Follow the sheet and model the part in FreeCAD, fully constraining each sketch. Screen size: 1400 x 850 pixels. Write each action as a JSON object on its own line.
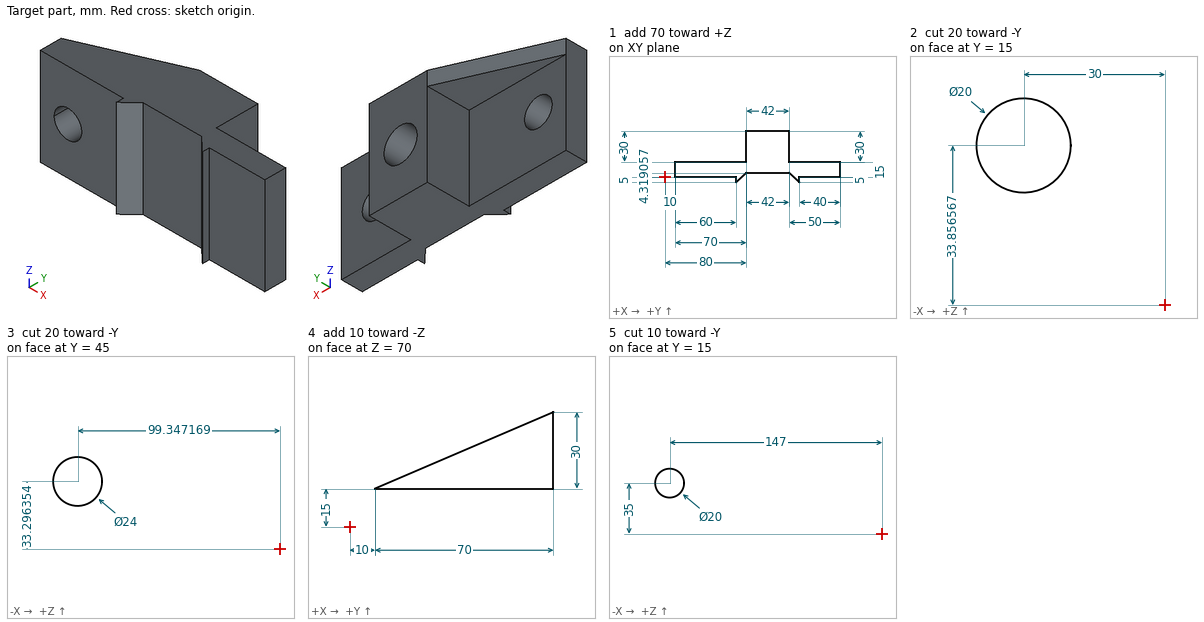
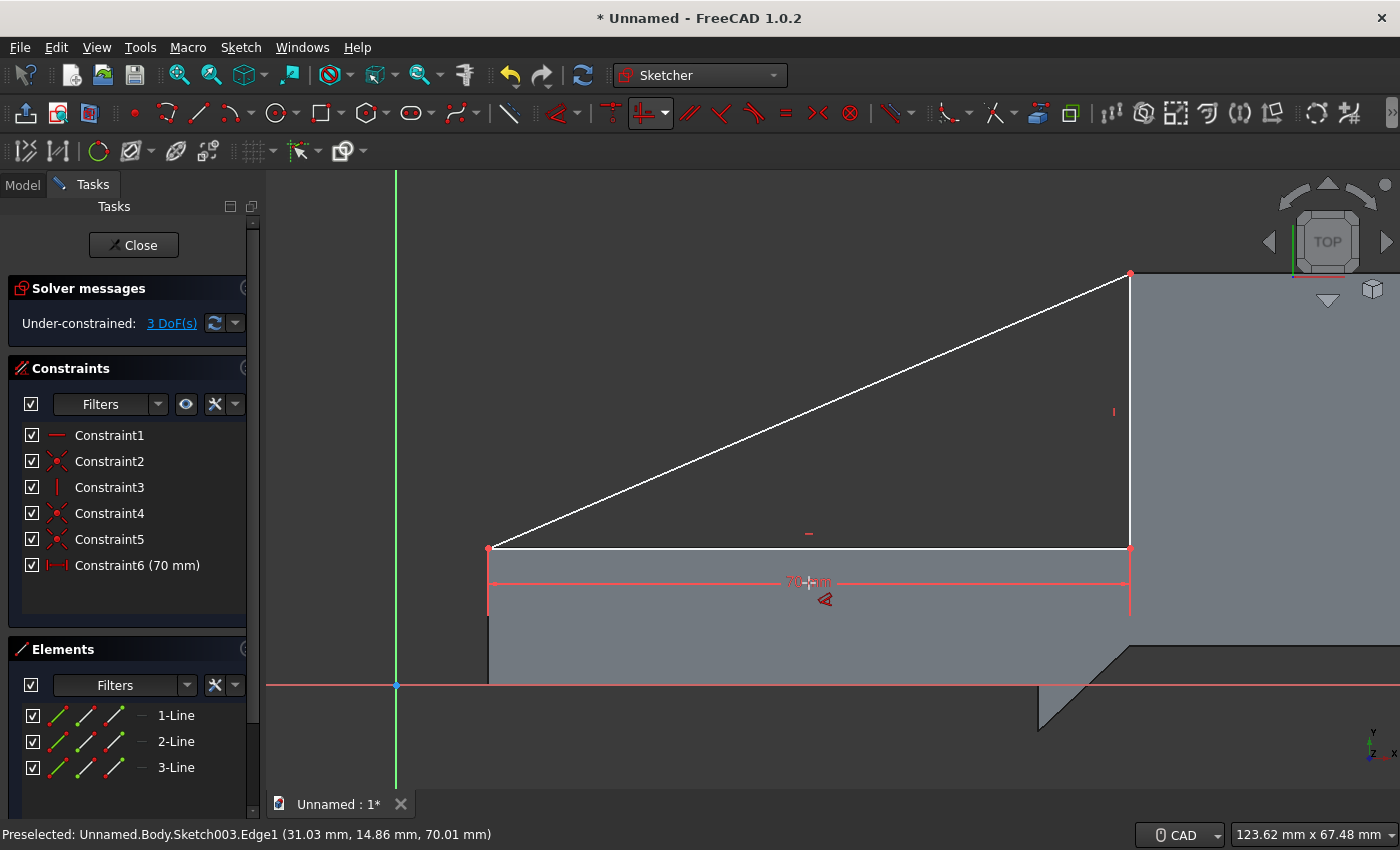
{"action": "left_click", "coordinate": [1130, 466]}
{"action": "left_click", "coordinate": [1164, 411]}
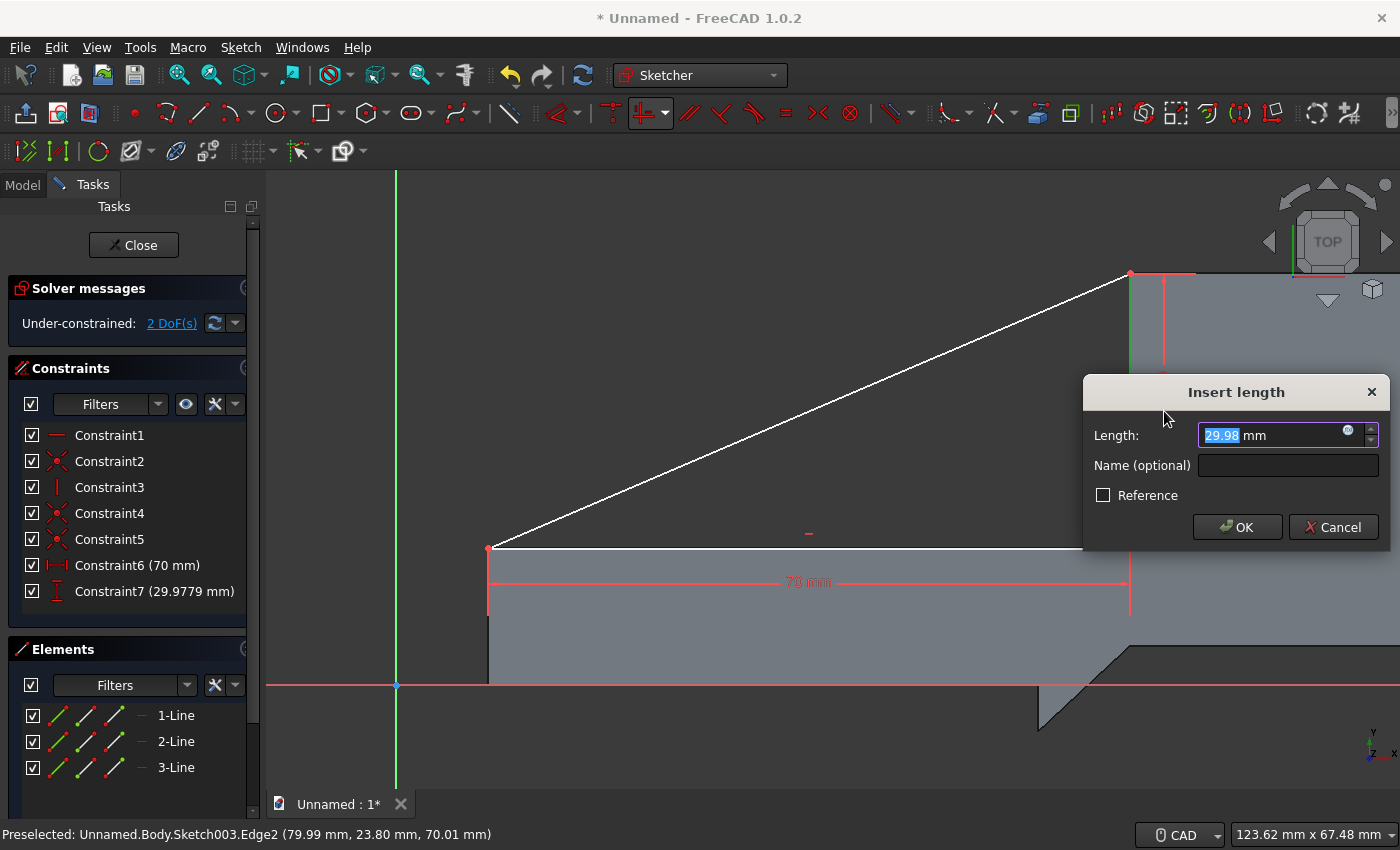
{"action": "type", "text": "30"}
{"action": "key", "text": "Return"}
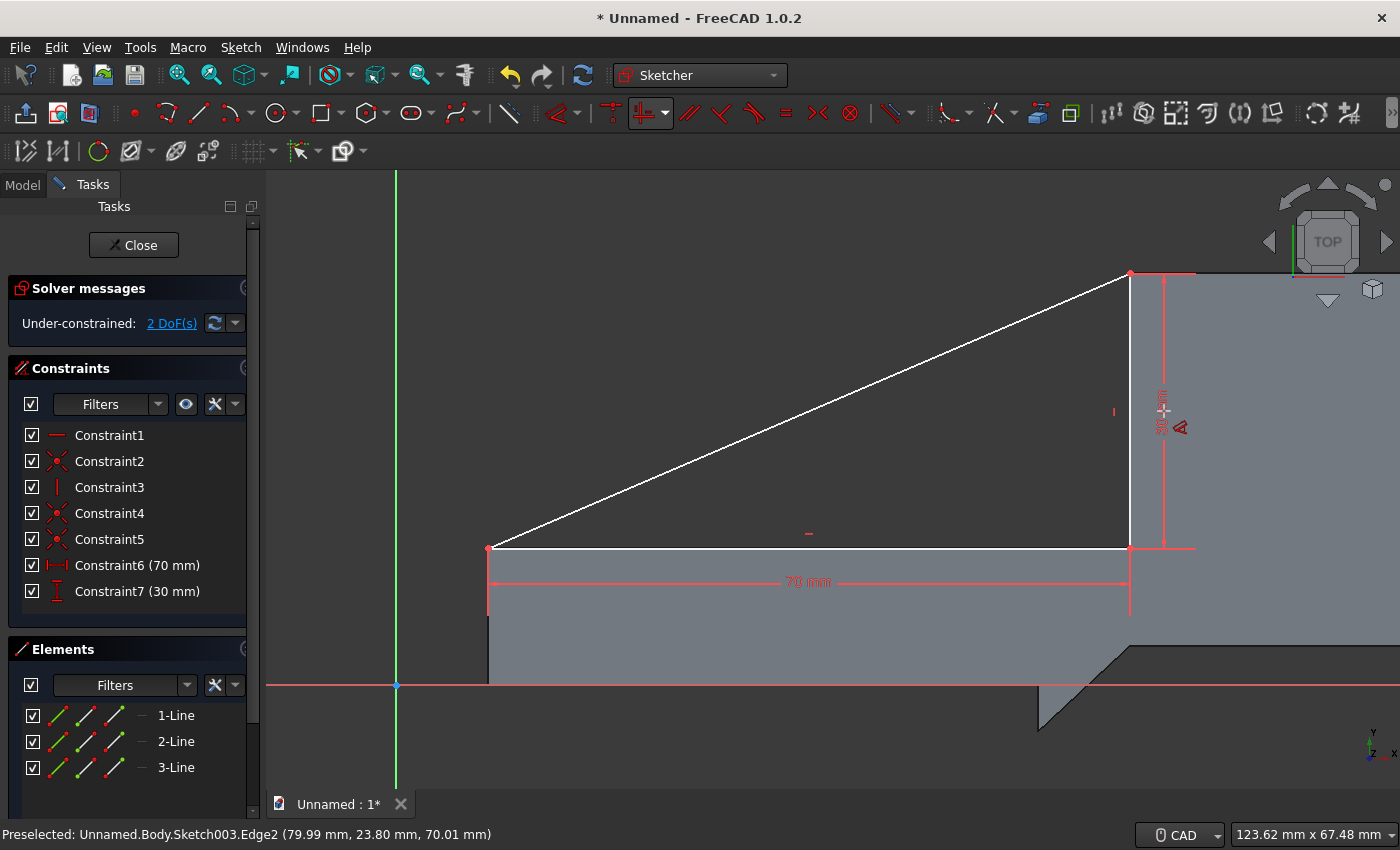
{"action": "left_click", "coordinate": [488, 549]}
{"action": "left_click", "coordinate": [442, 719]}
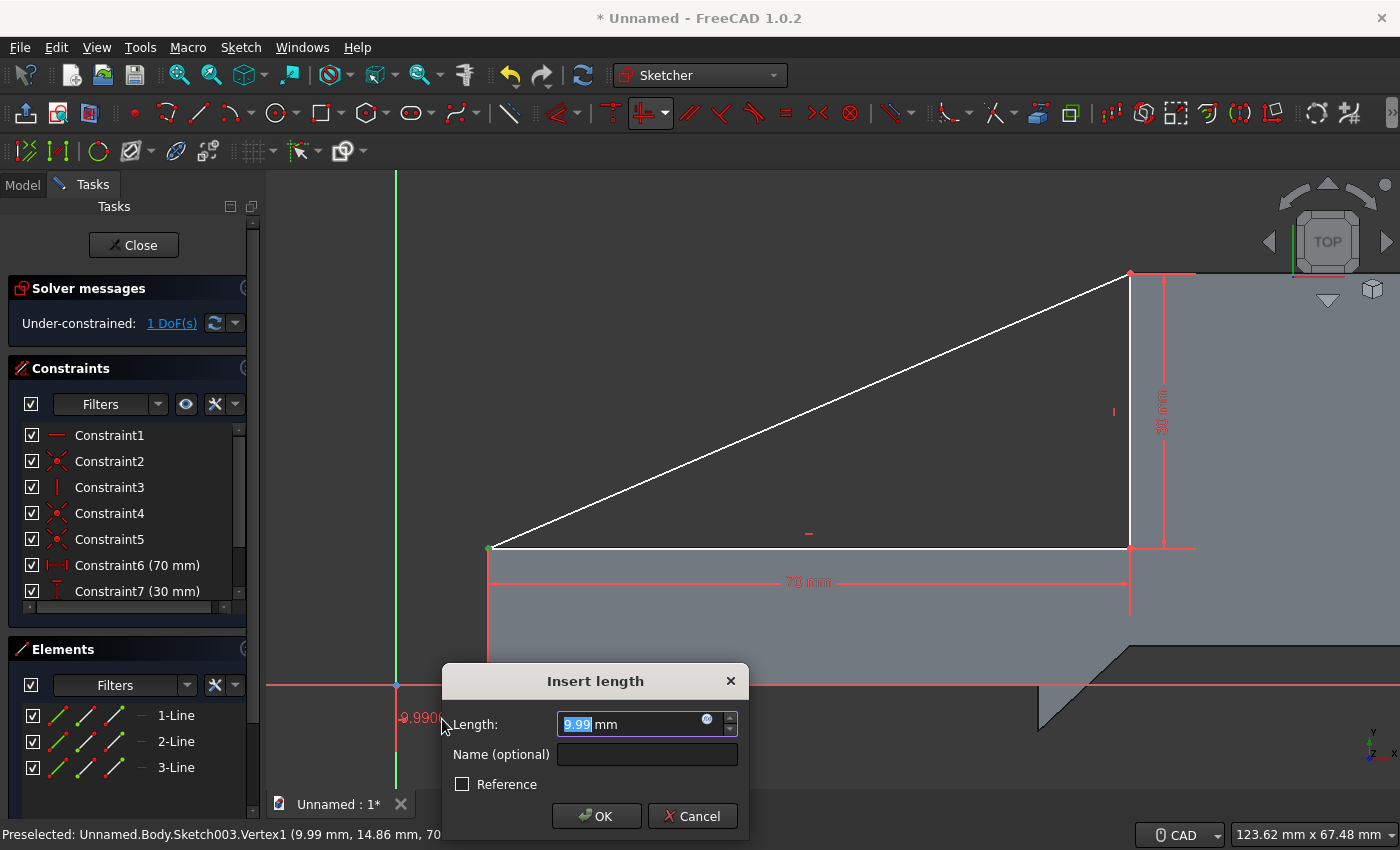
{"action": "type", "text": "10"}
{"action": "key", "text": "Return"}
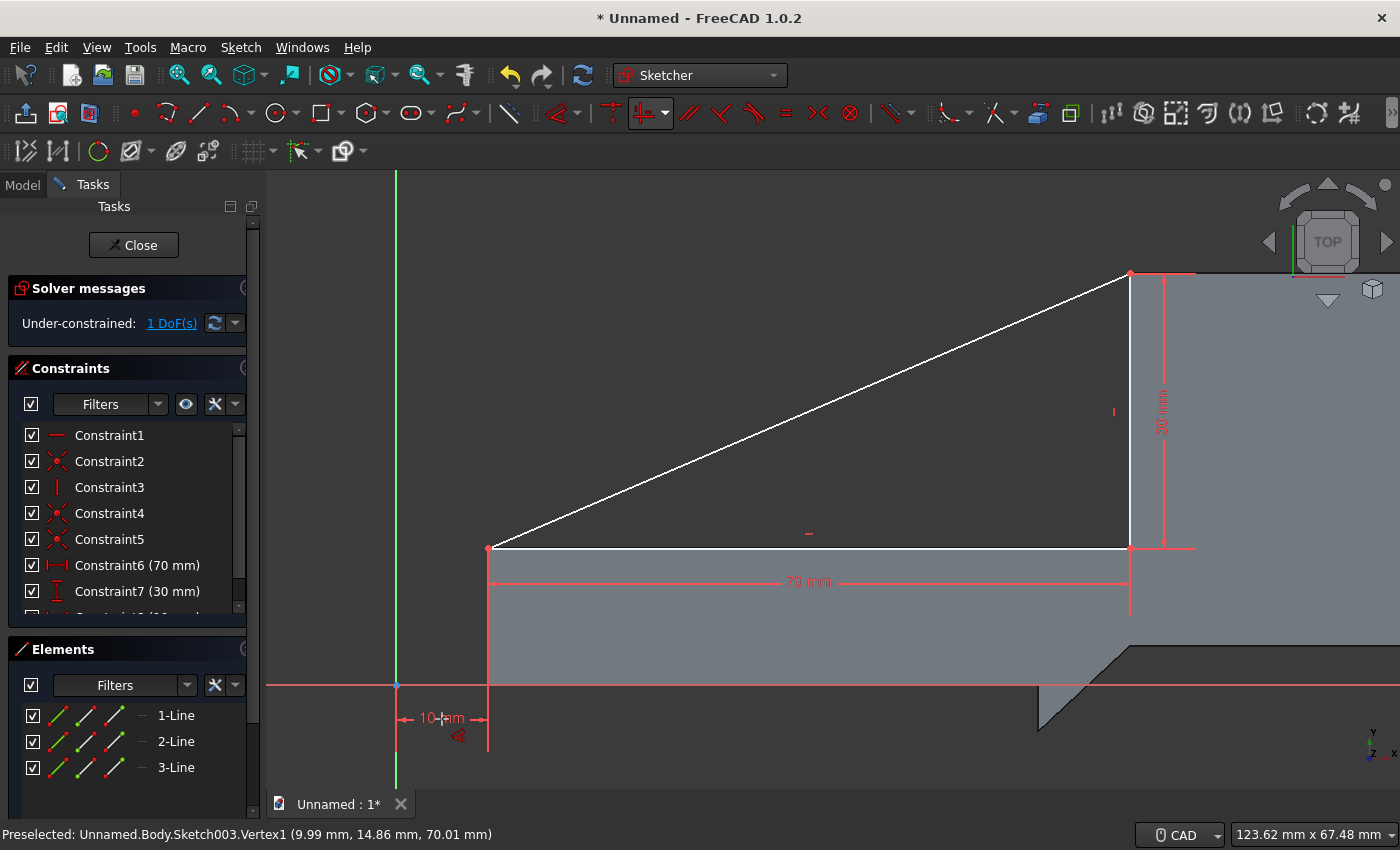
{"action": "left_click", "coordinate": [488, 549]}
{"action": "left_click", "coordinate": [362, 617]}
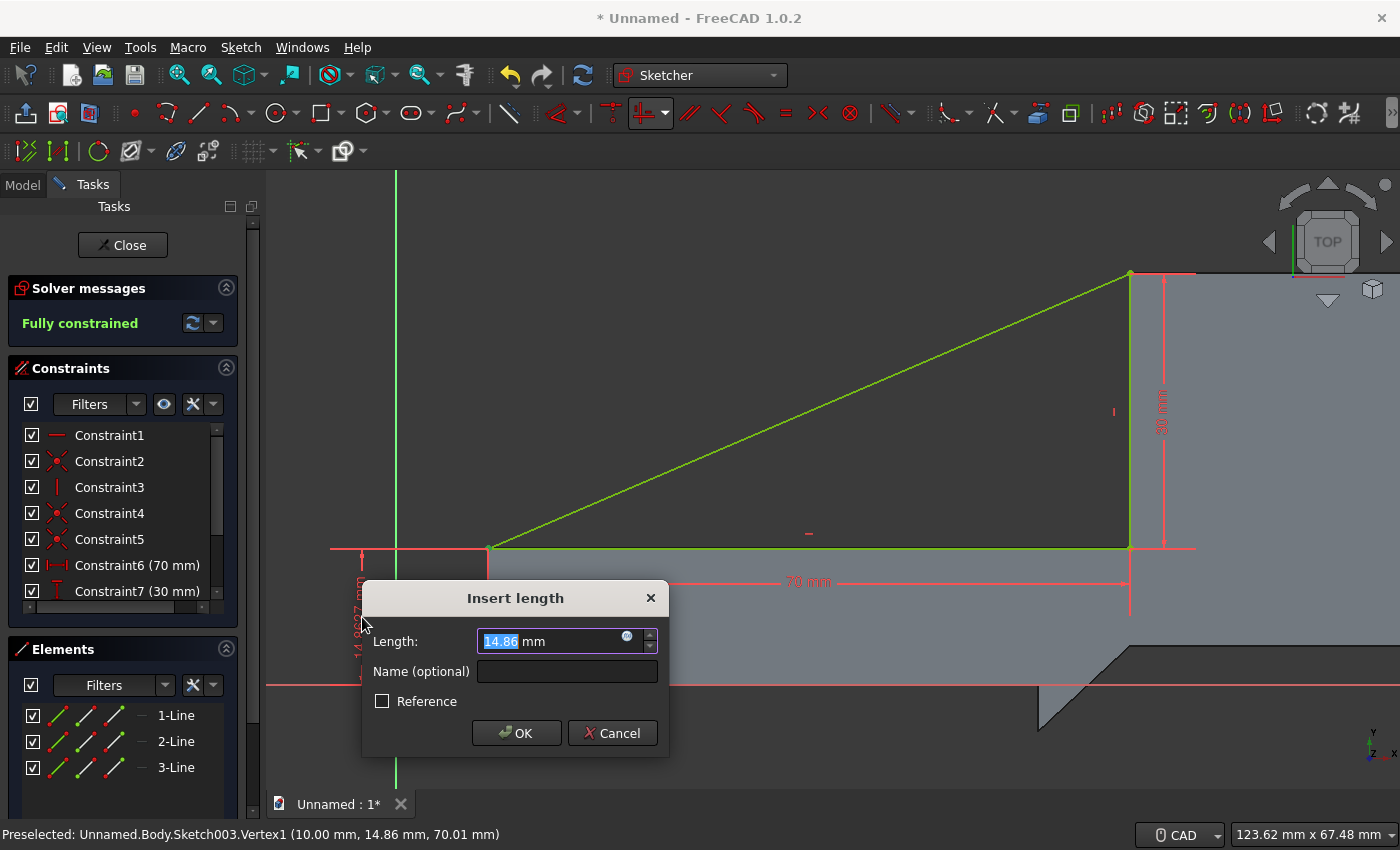
{"action": "type", "text": "15"}
{"action": "key", "text": "Return"}
{"action": "key", "text": "Escape"}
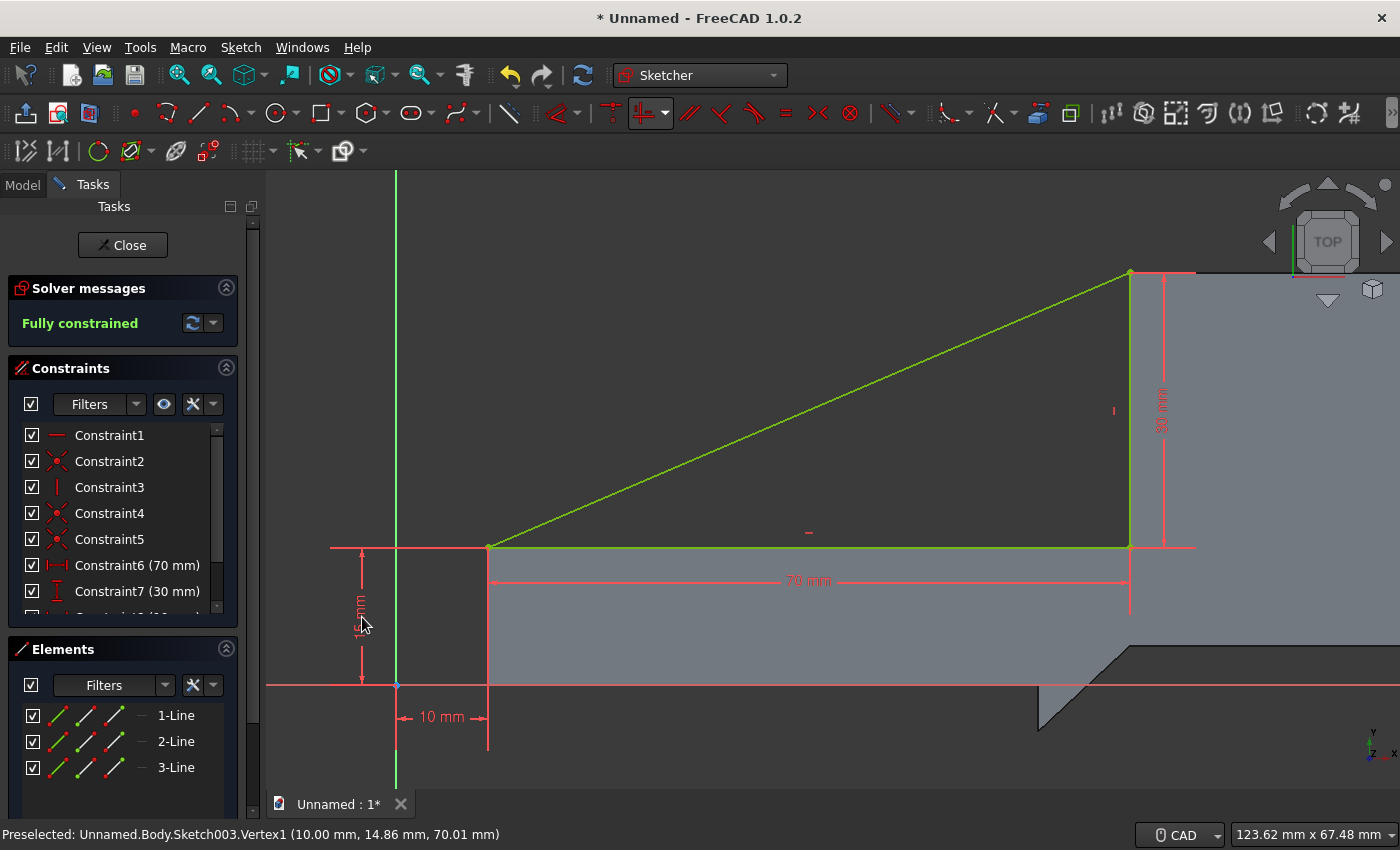
{"action": "left_click", "coordinate": [123, 245]}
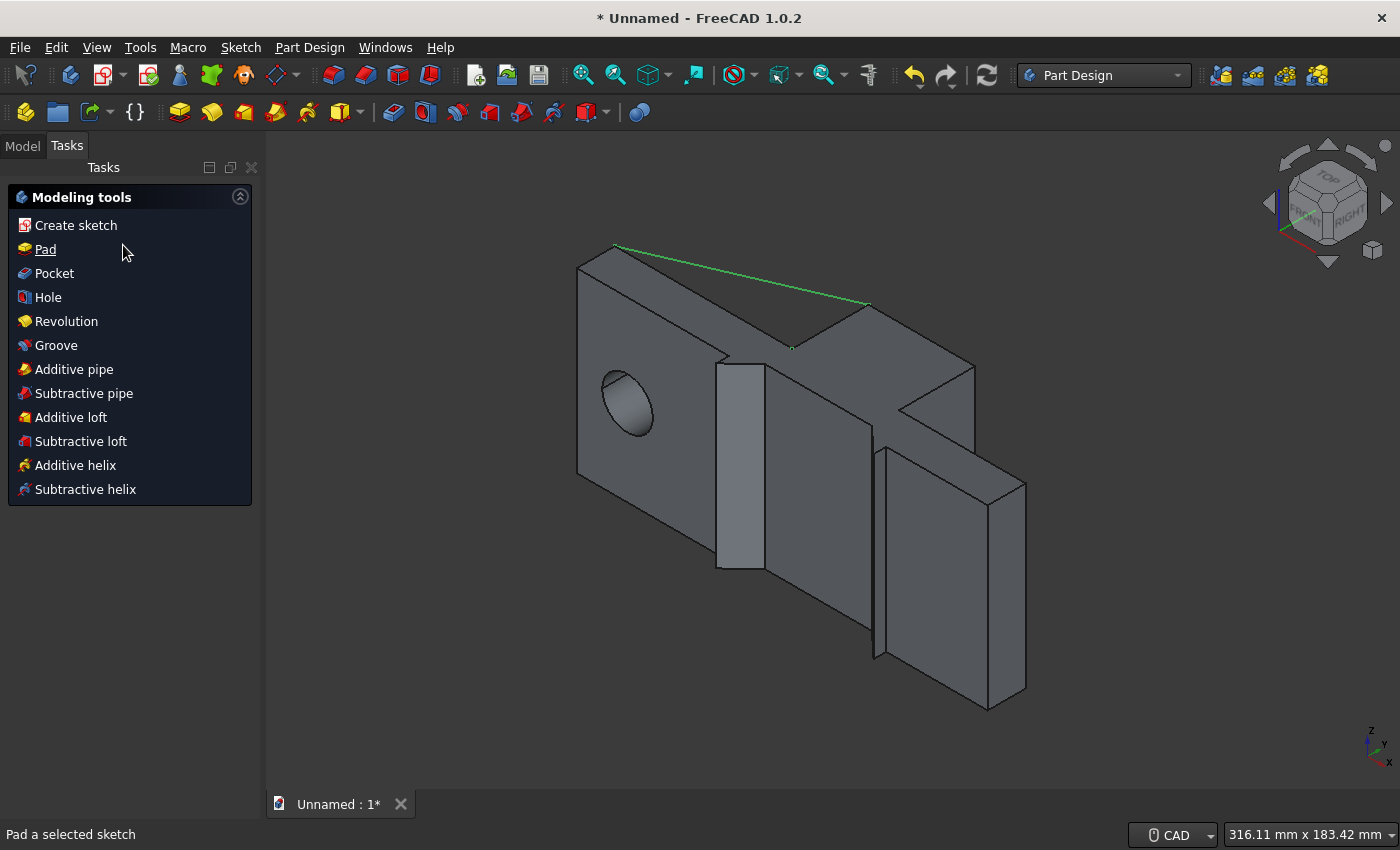
{"action": "left_click", "coordinate": [180, 112]}